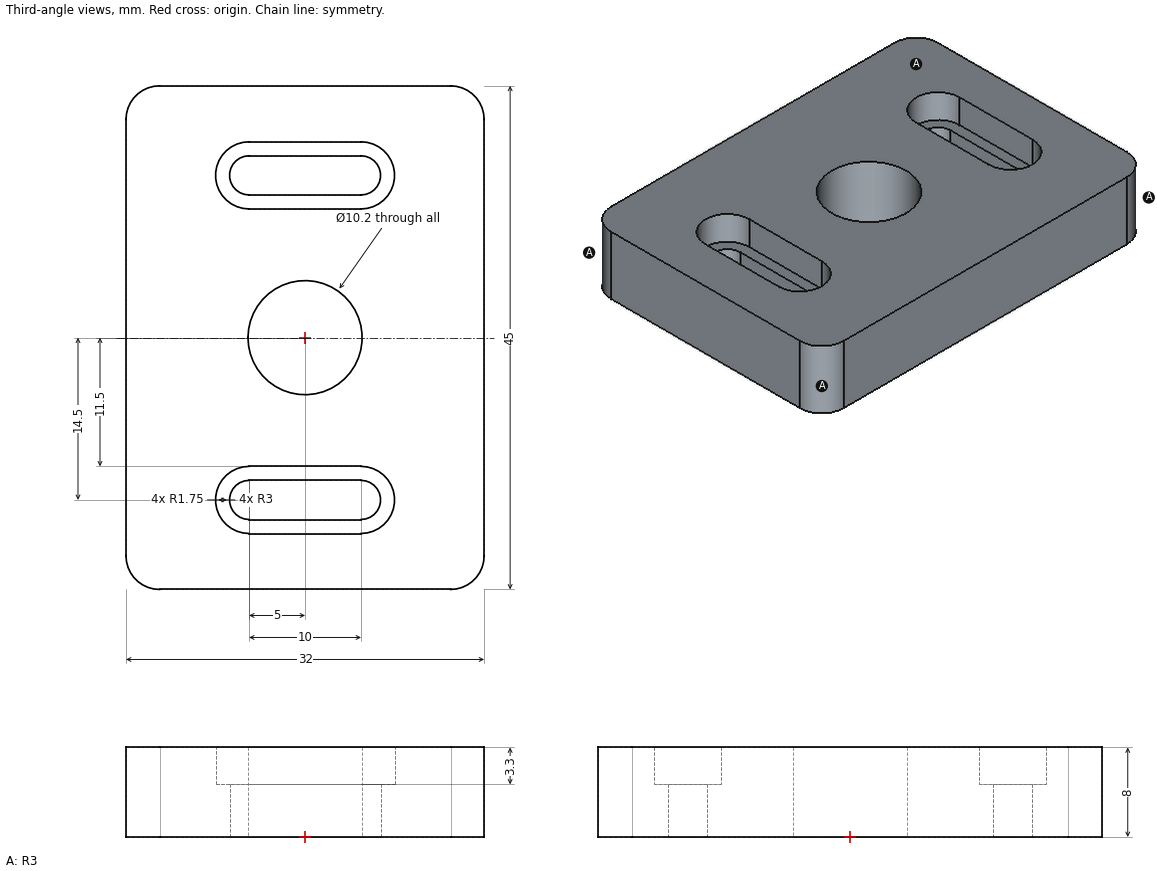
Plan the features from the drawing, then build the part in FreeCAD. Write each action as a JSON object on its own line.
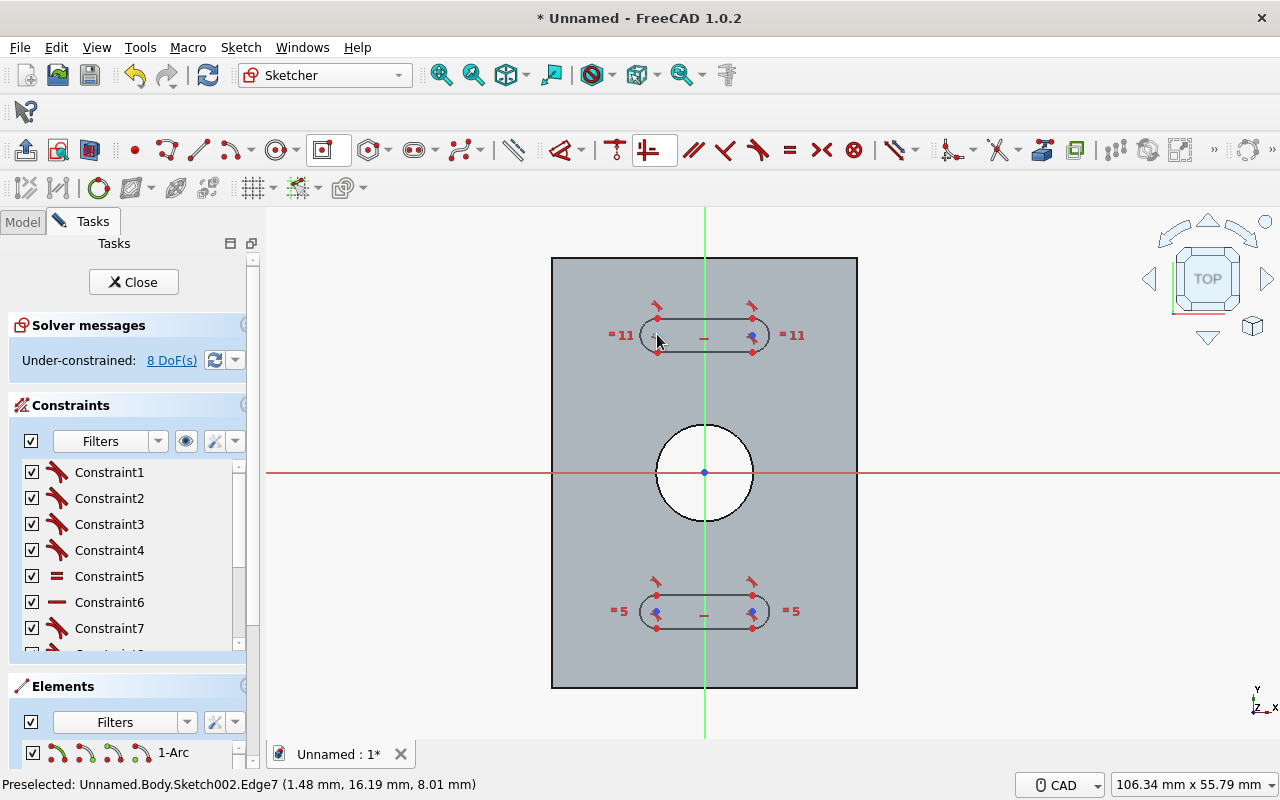
{"action": "left_click", "coordinate": [643, 602]}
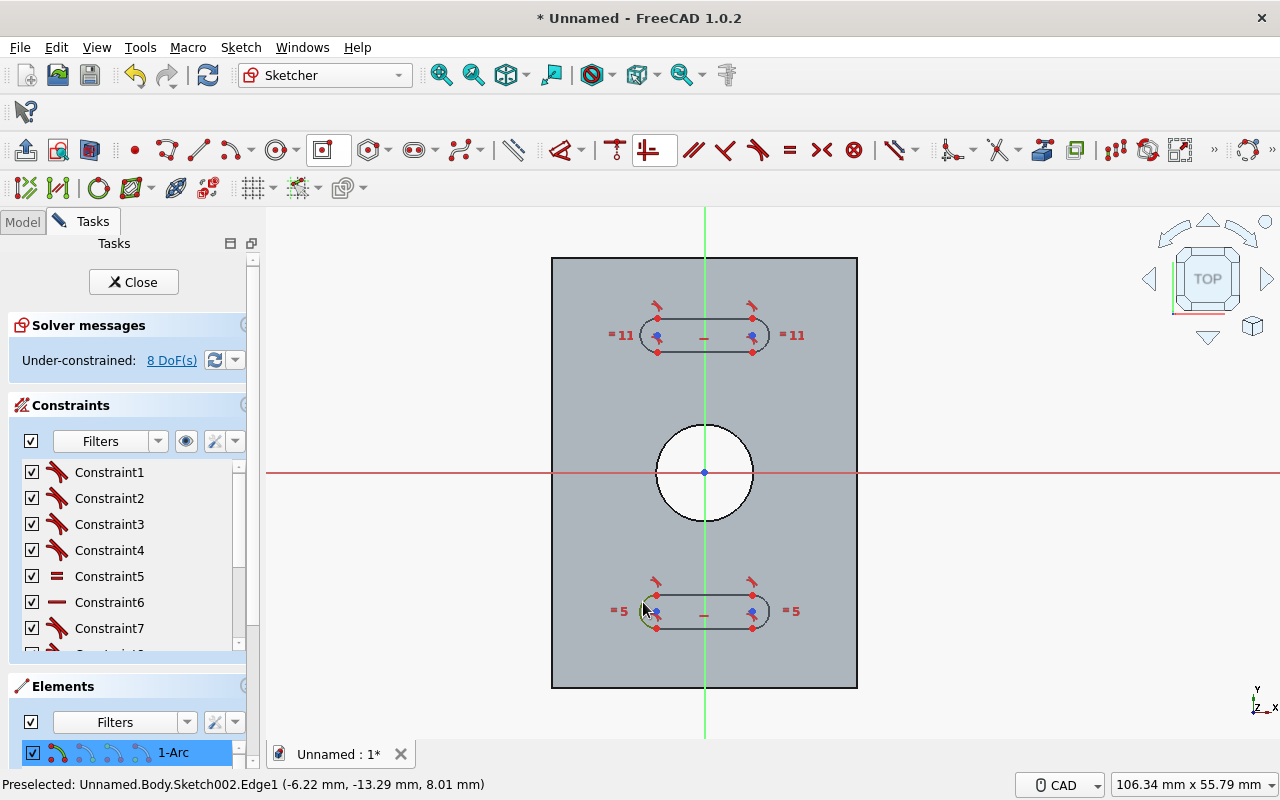
{"action": "left_click", "coordinate": [644, 326]}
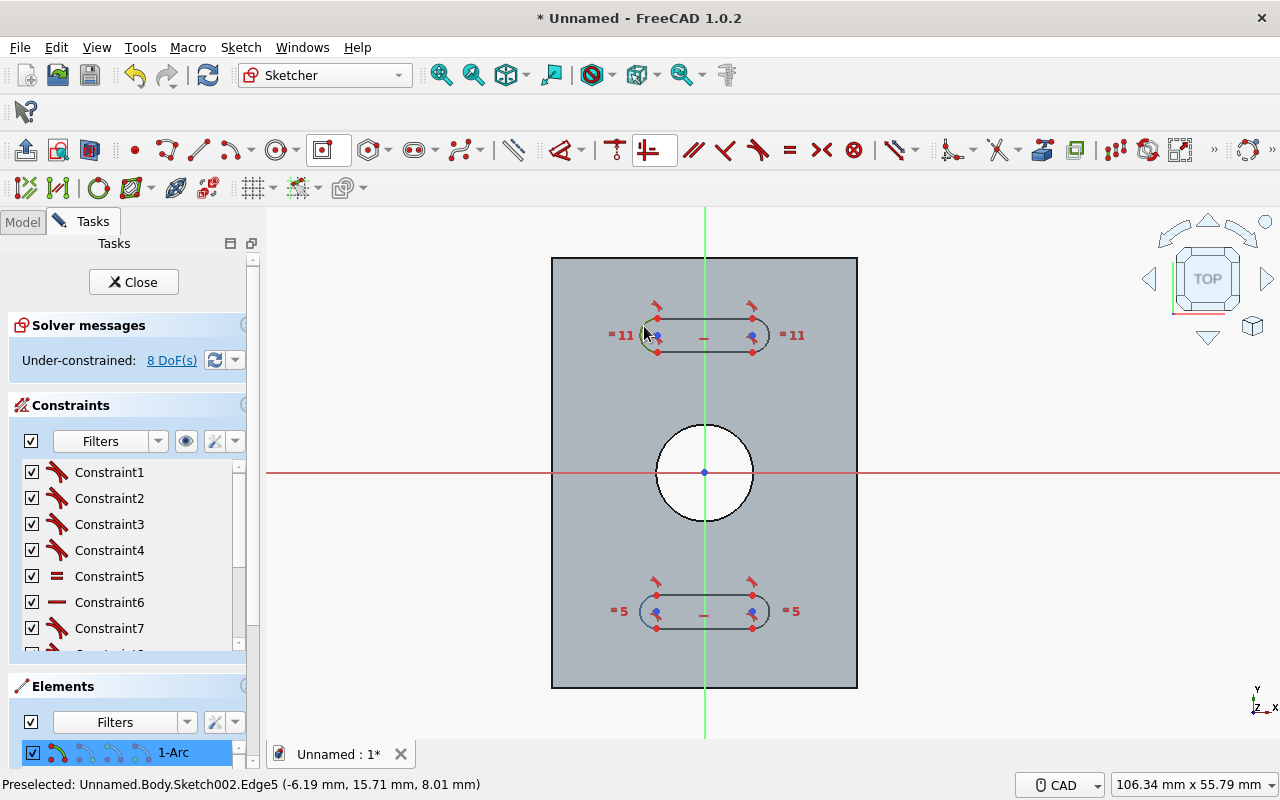
{"action": "left_click", "coordinate": [790, 150]}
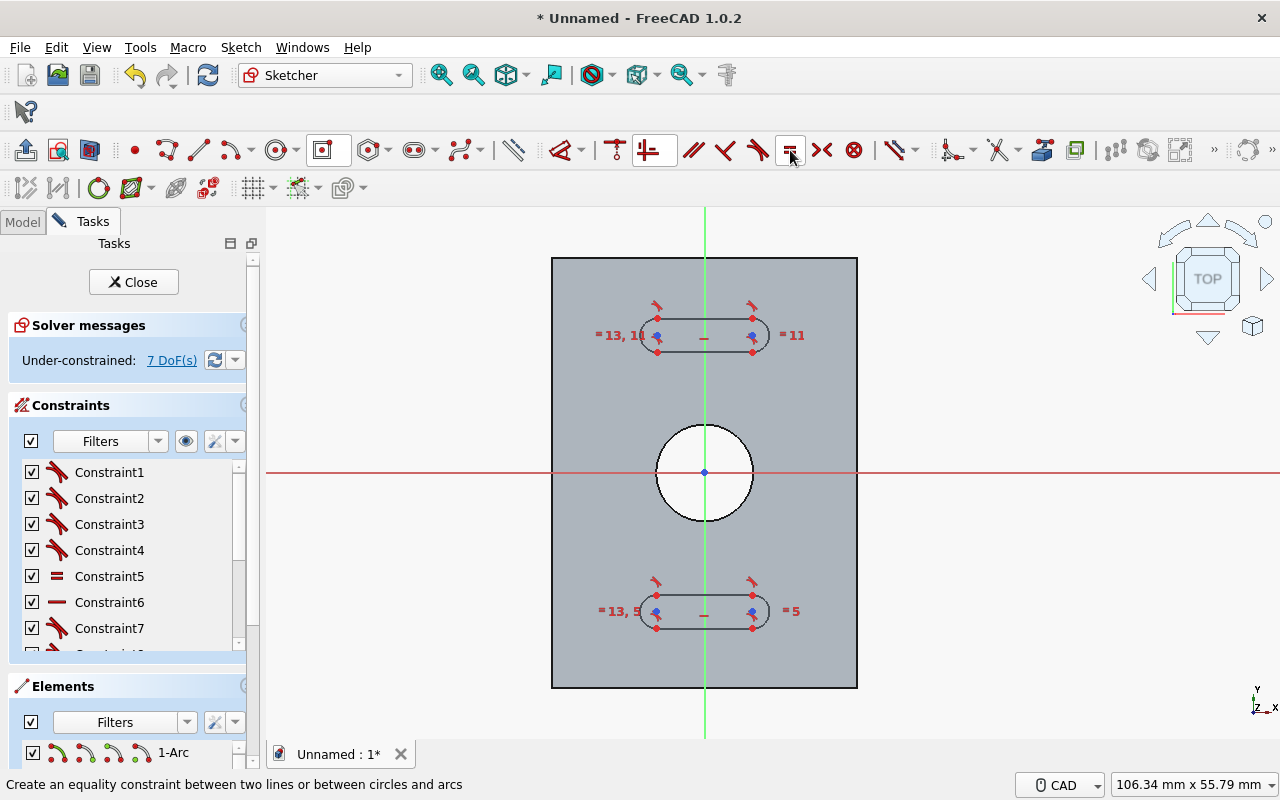
{"action": "left_click", "coordinate": [657, 612]}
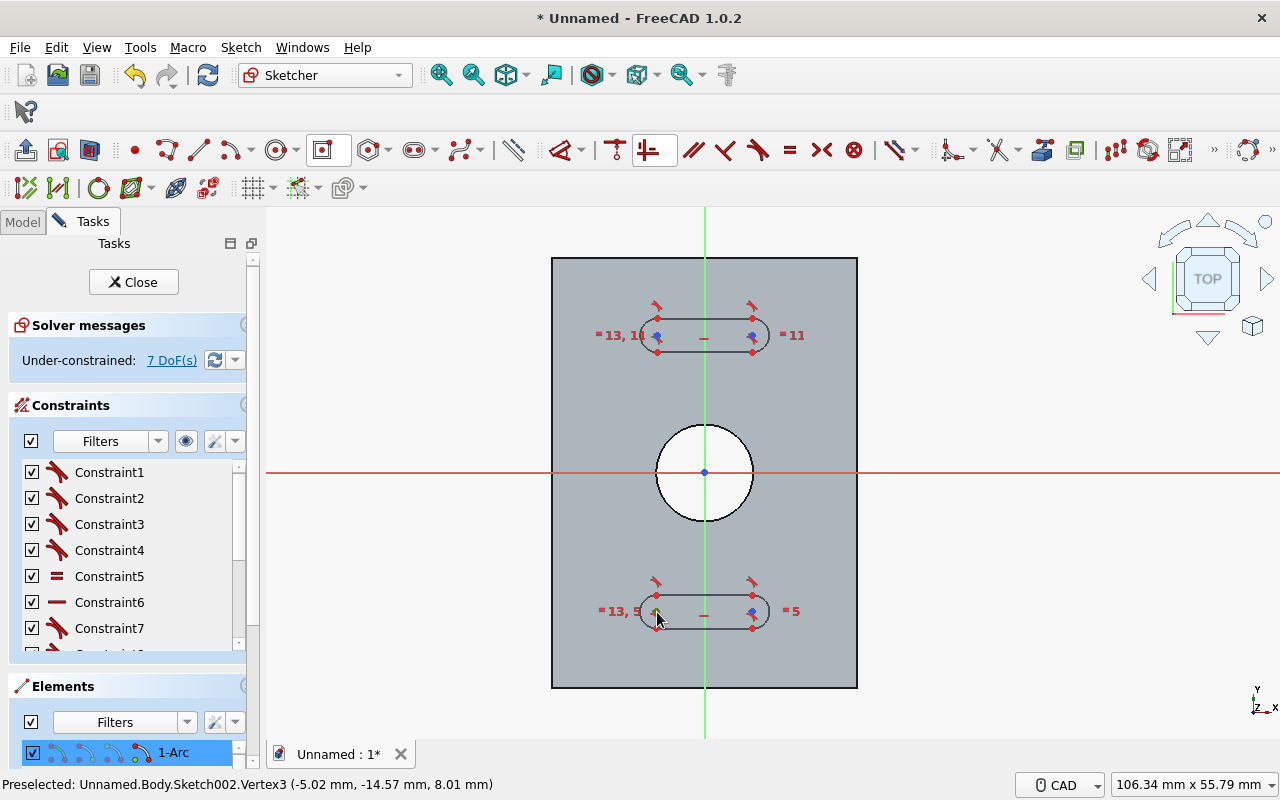
{"action": "left_click", "coordinate": [657, 335]}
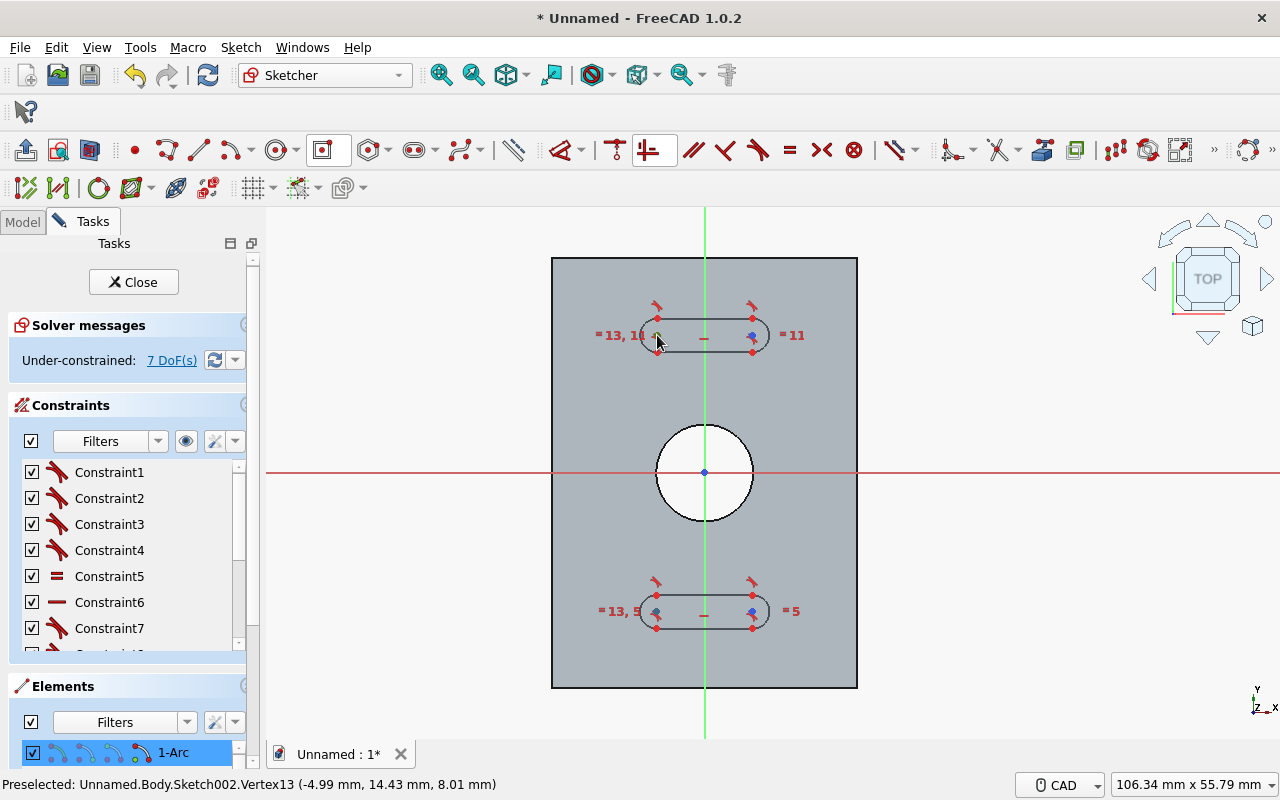
{"action": "left_click", "coordinate": [353, 473]}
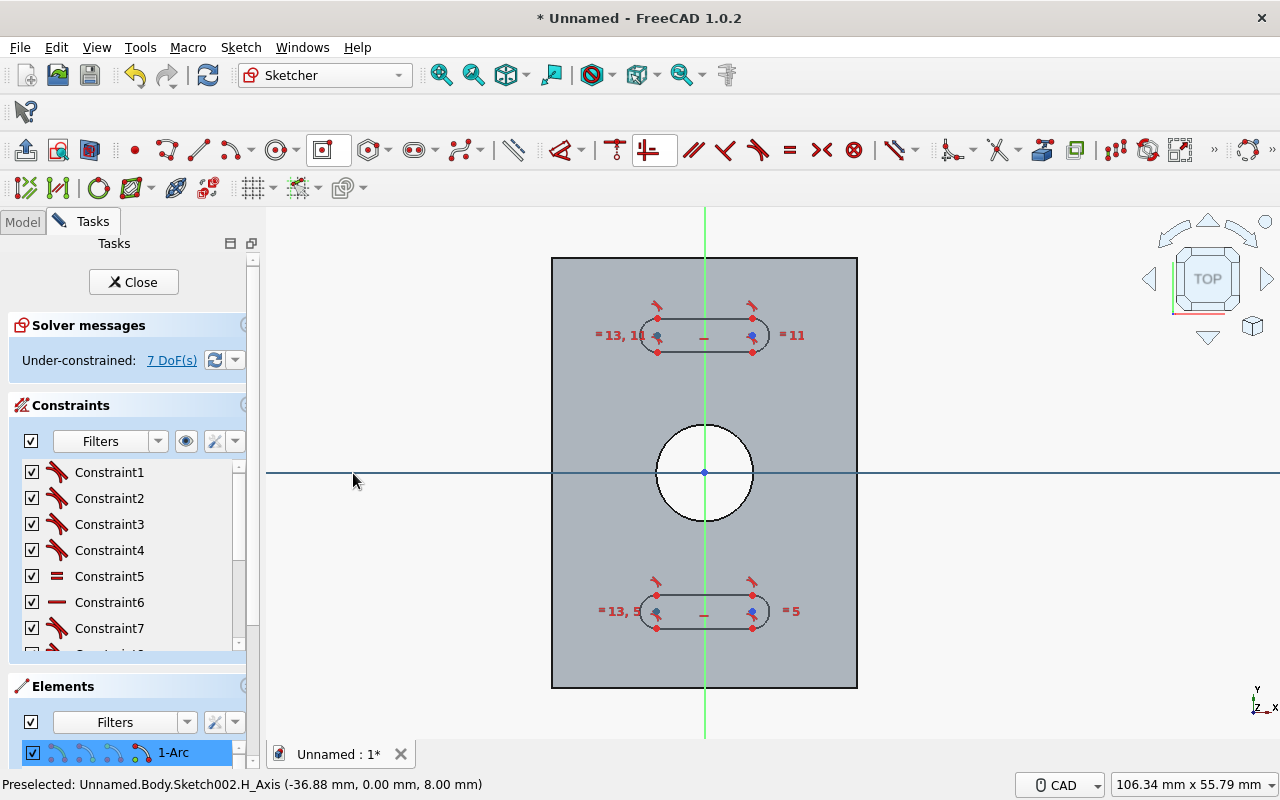
{"action": "left_click", "coordinate": [822, 150]}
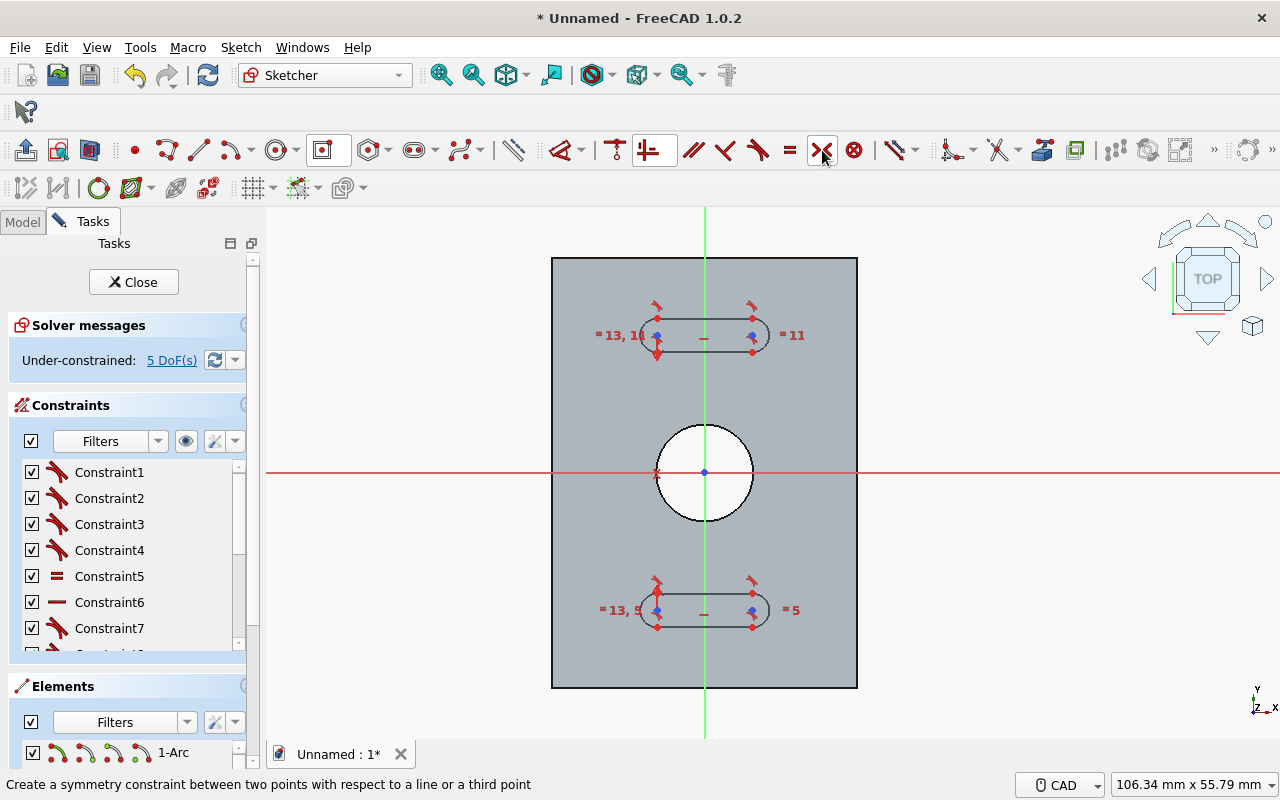
{"action": "left_click", "coordinate": [560, 150]}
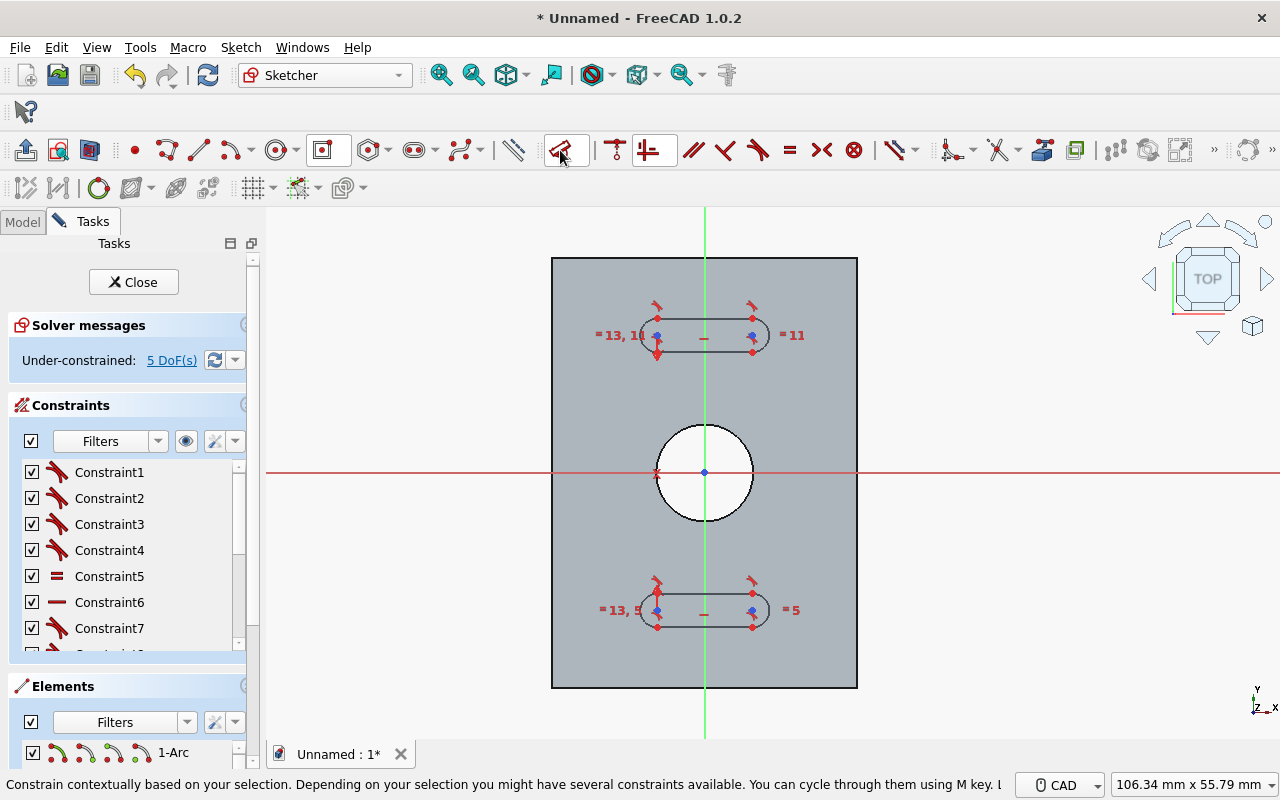
{"action": "scroll", "coordinate": [644, 601], "scroll_direction": "up", "scroll_amount": 5}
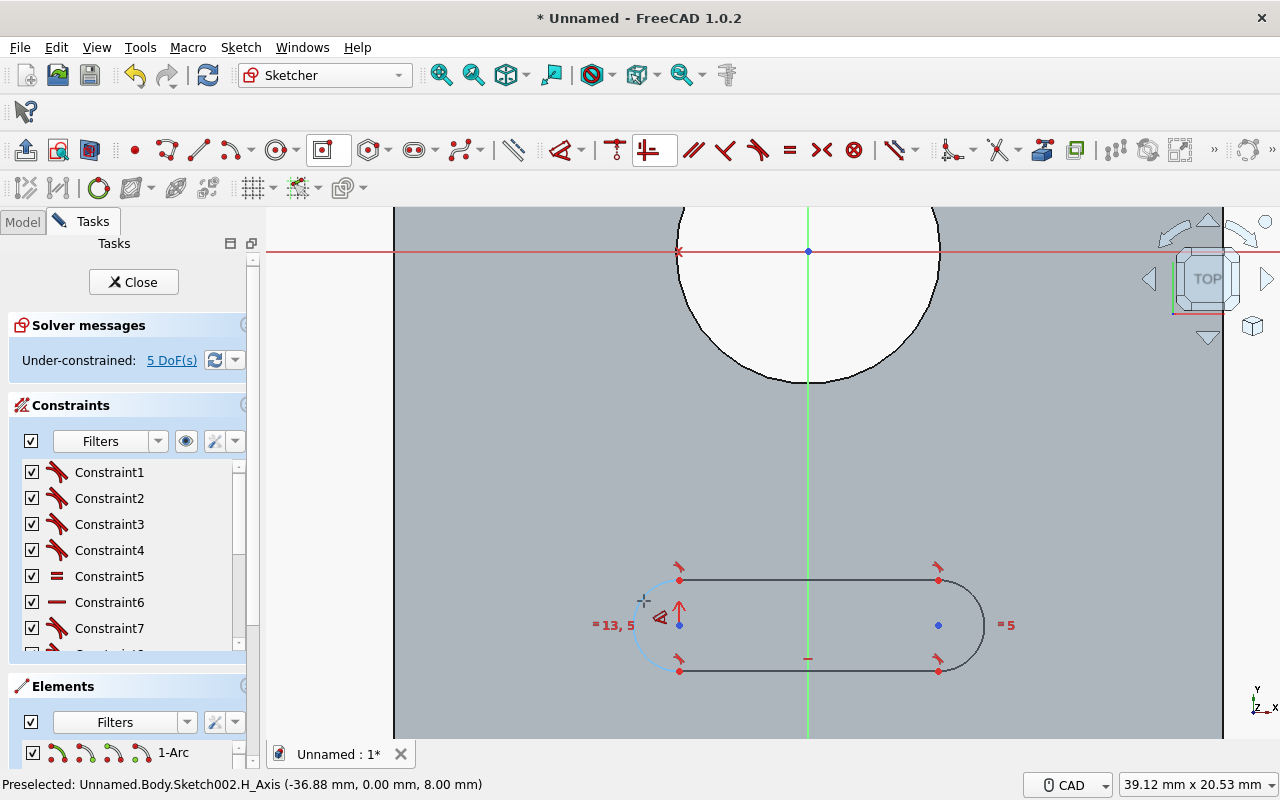
{"action": "left_click", "coordinate": [642, 599]}
{"action": "left_click", "coordinate": [616, 580]}